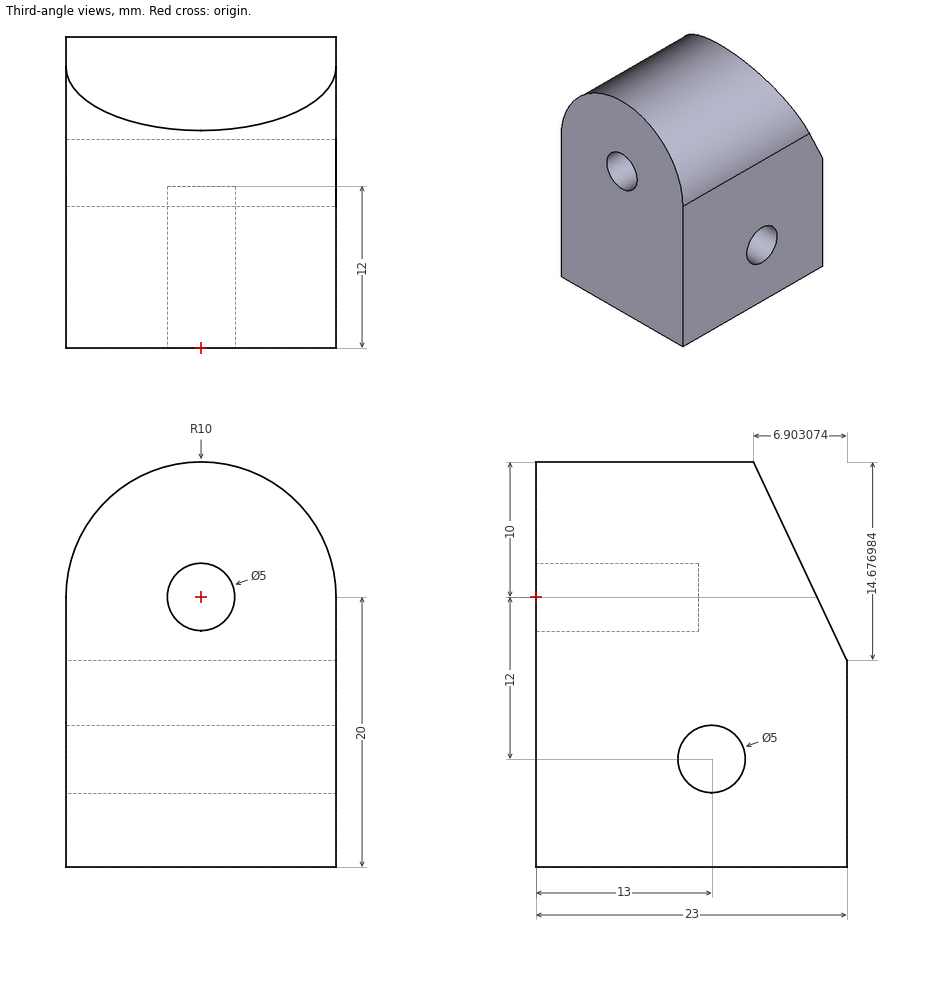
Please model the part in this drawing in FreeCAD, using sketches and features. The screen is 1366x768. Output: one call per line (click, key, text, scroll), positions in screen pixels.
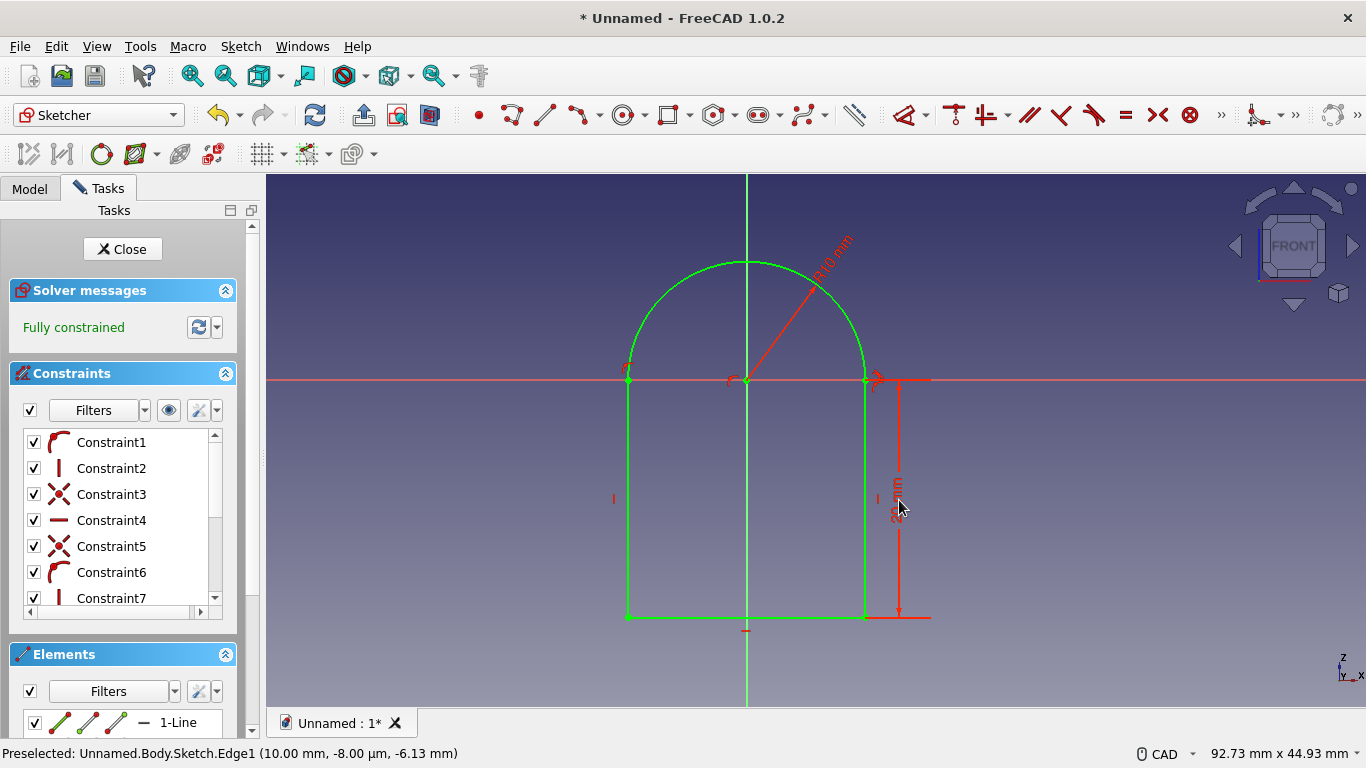
click(123, 249)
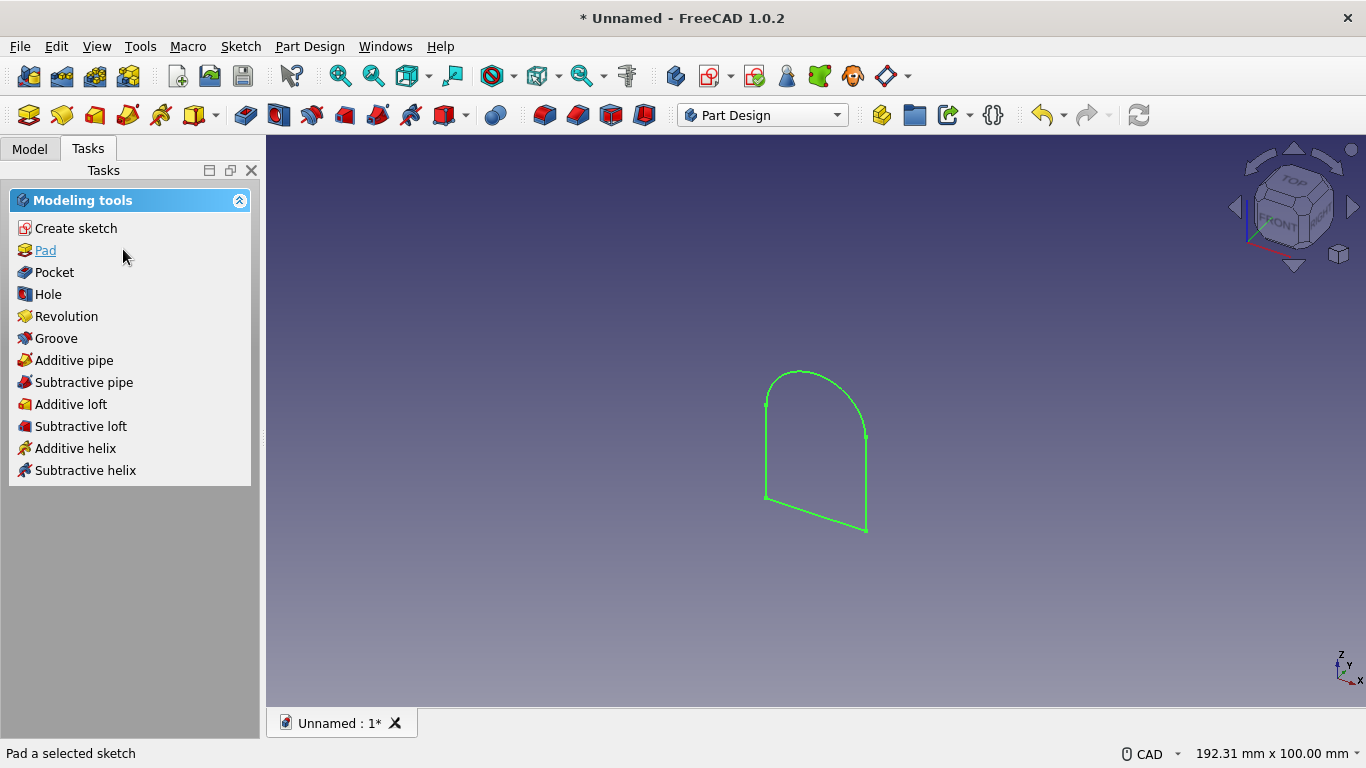
click(29, 116)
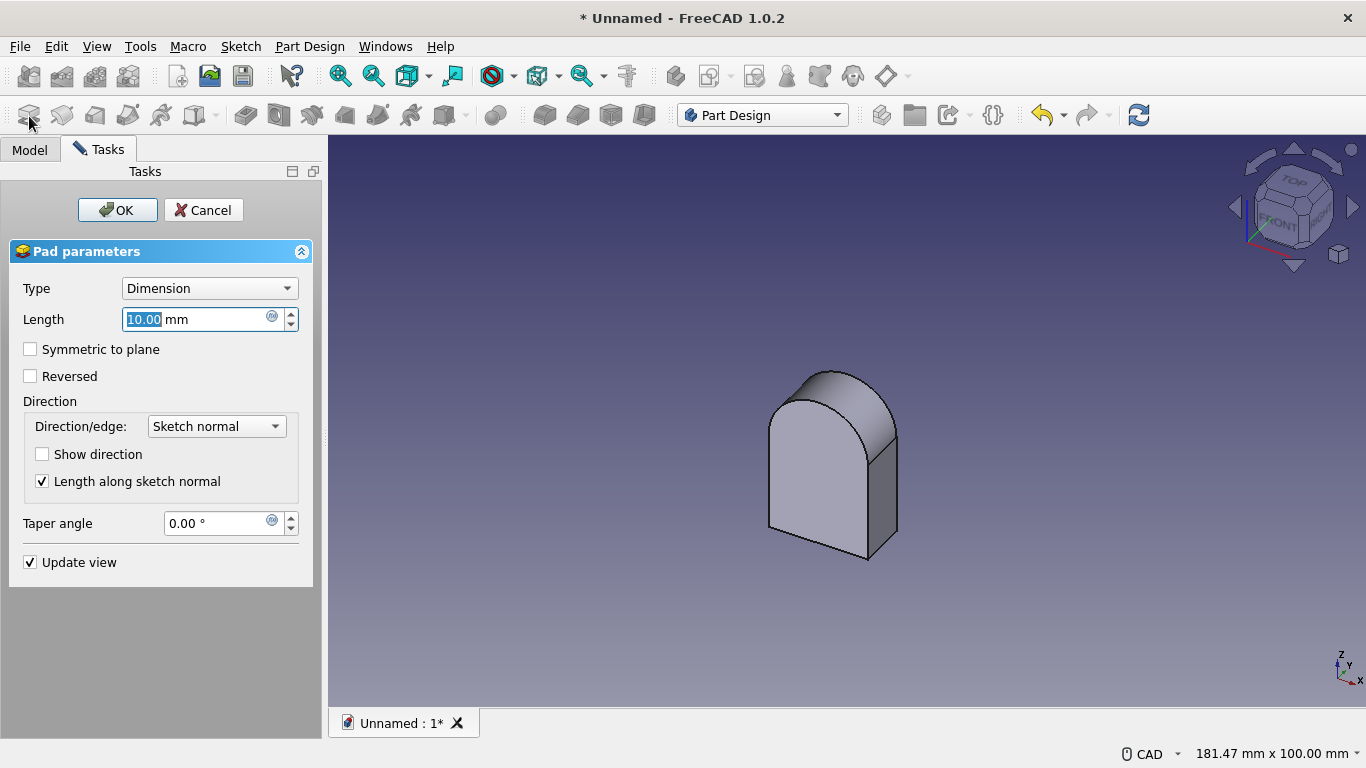
text(23)
key(Tab)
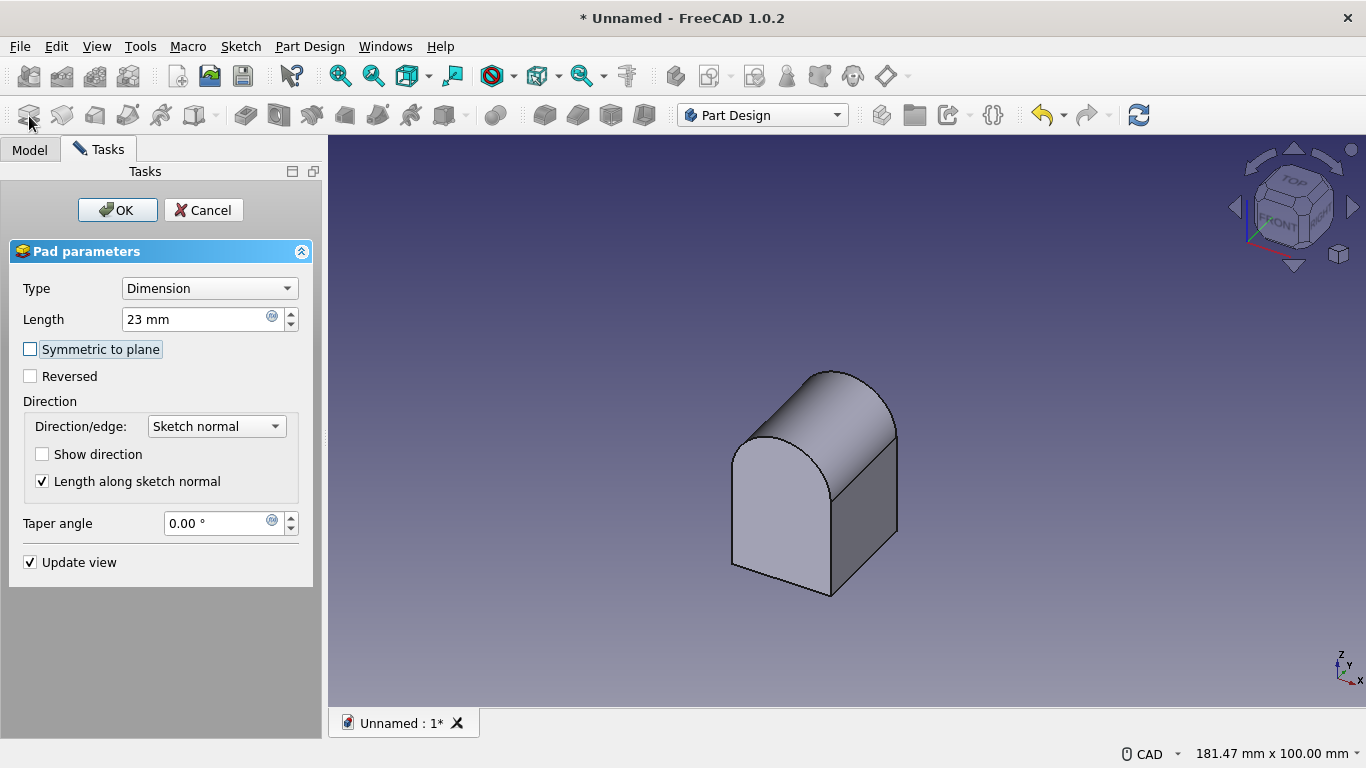
click(31, 376)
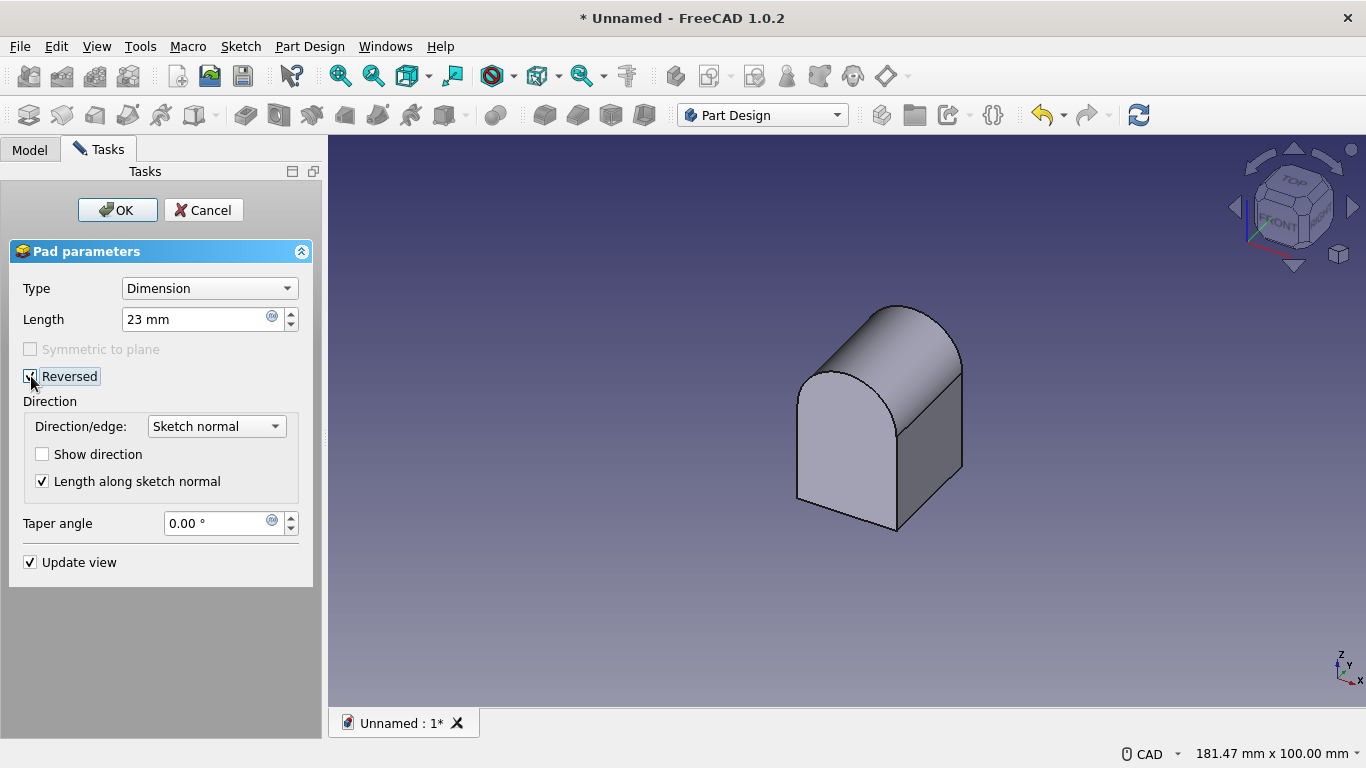
click(118, 210)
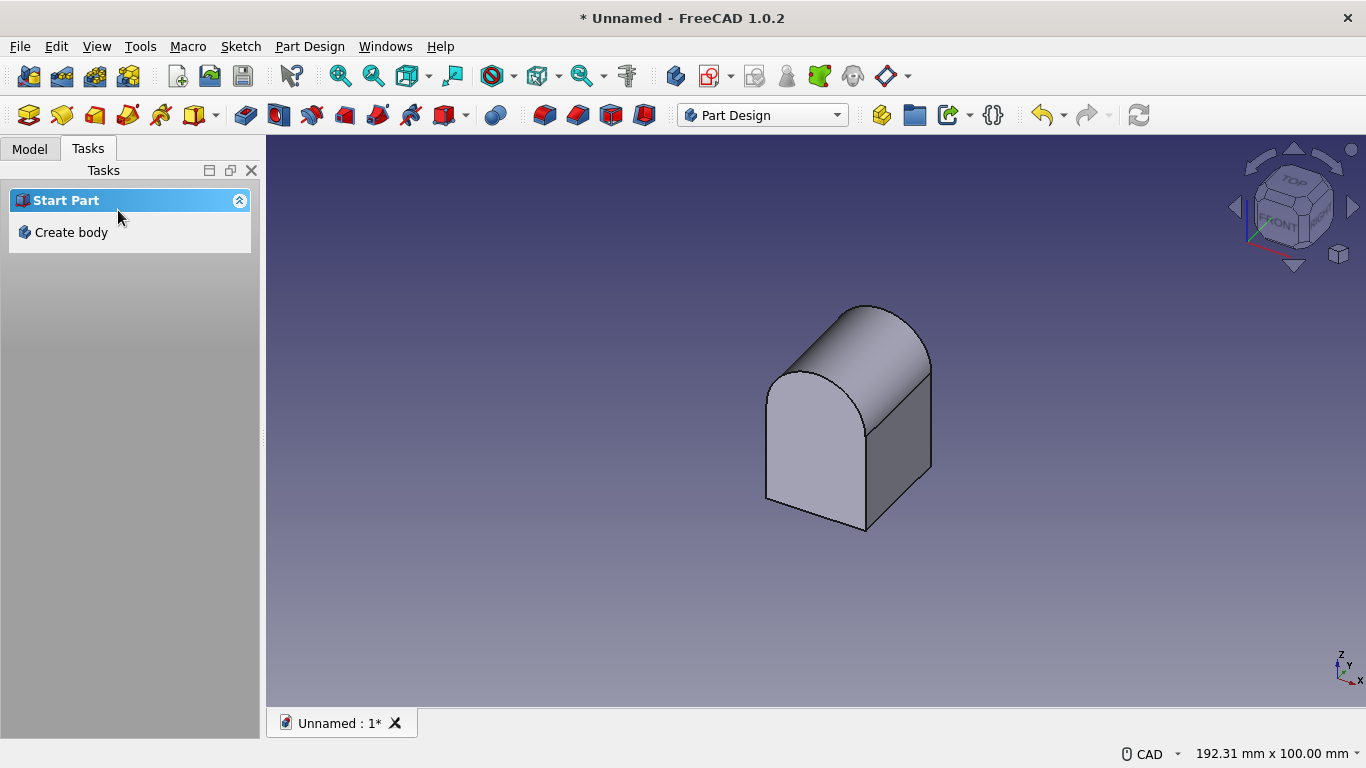
click(341, 76)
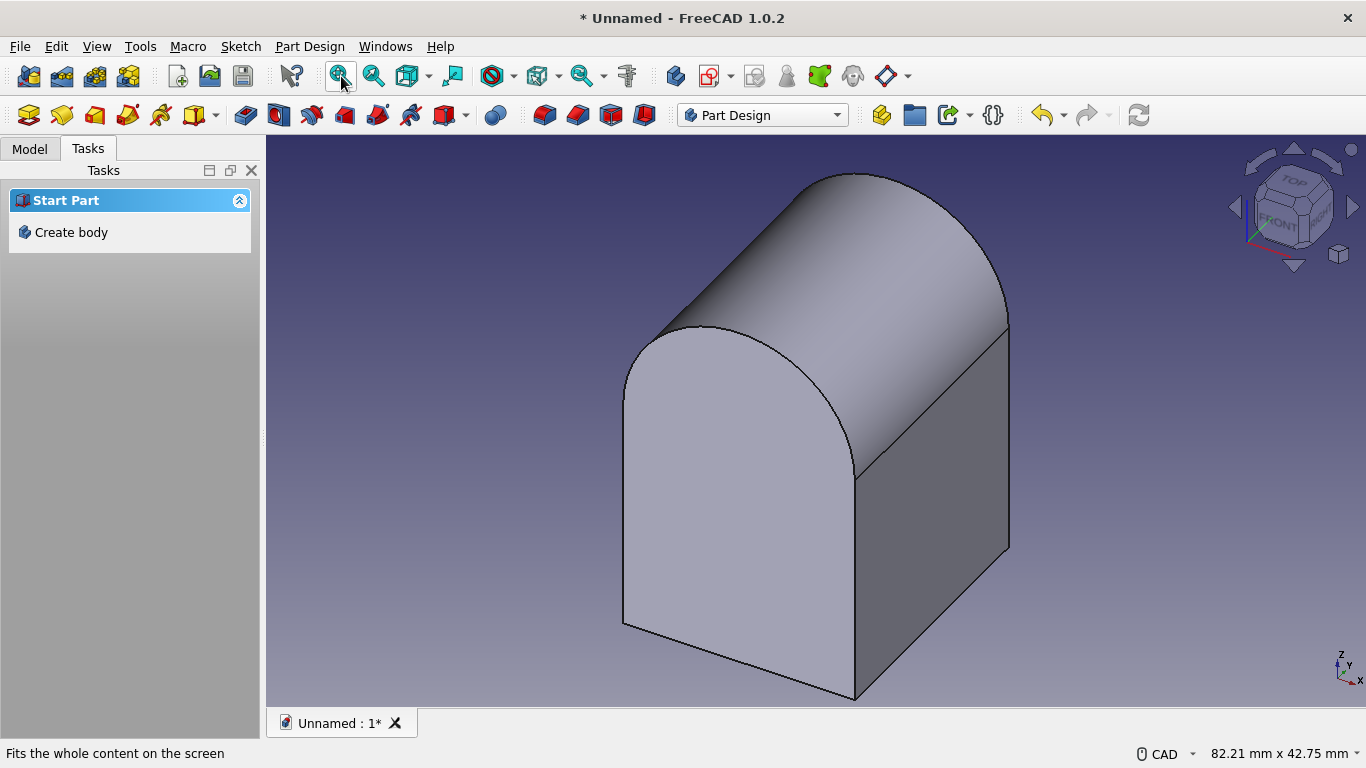
click(708, 76)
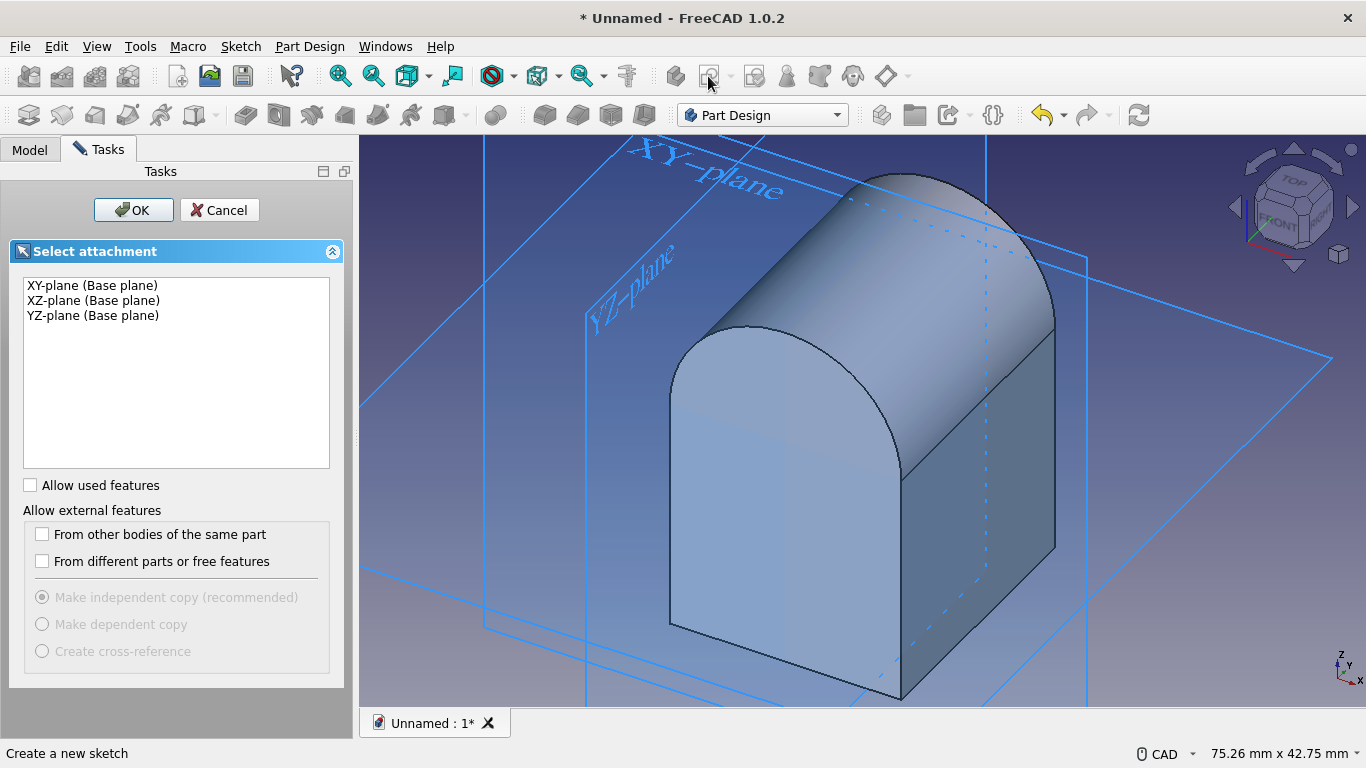
click(84, 300)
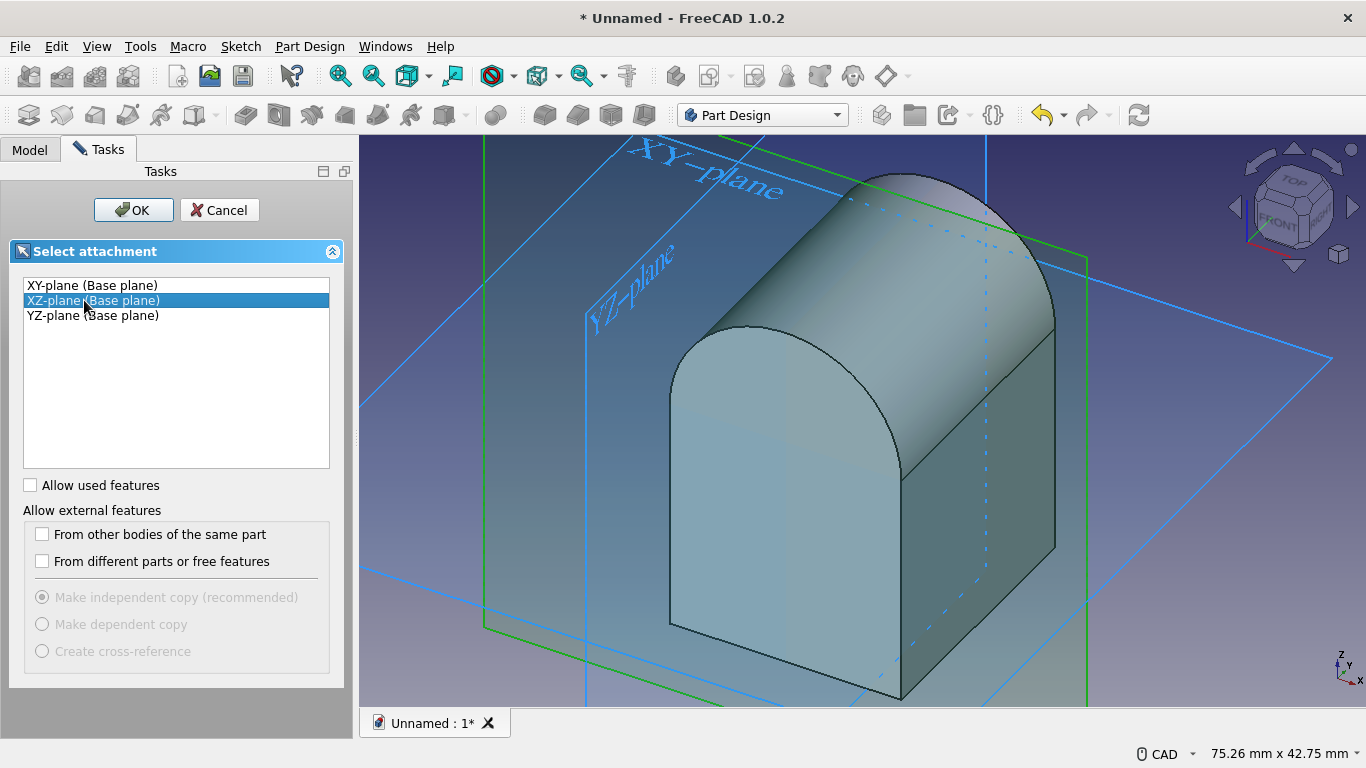
click(134, 210)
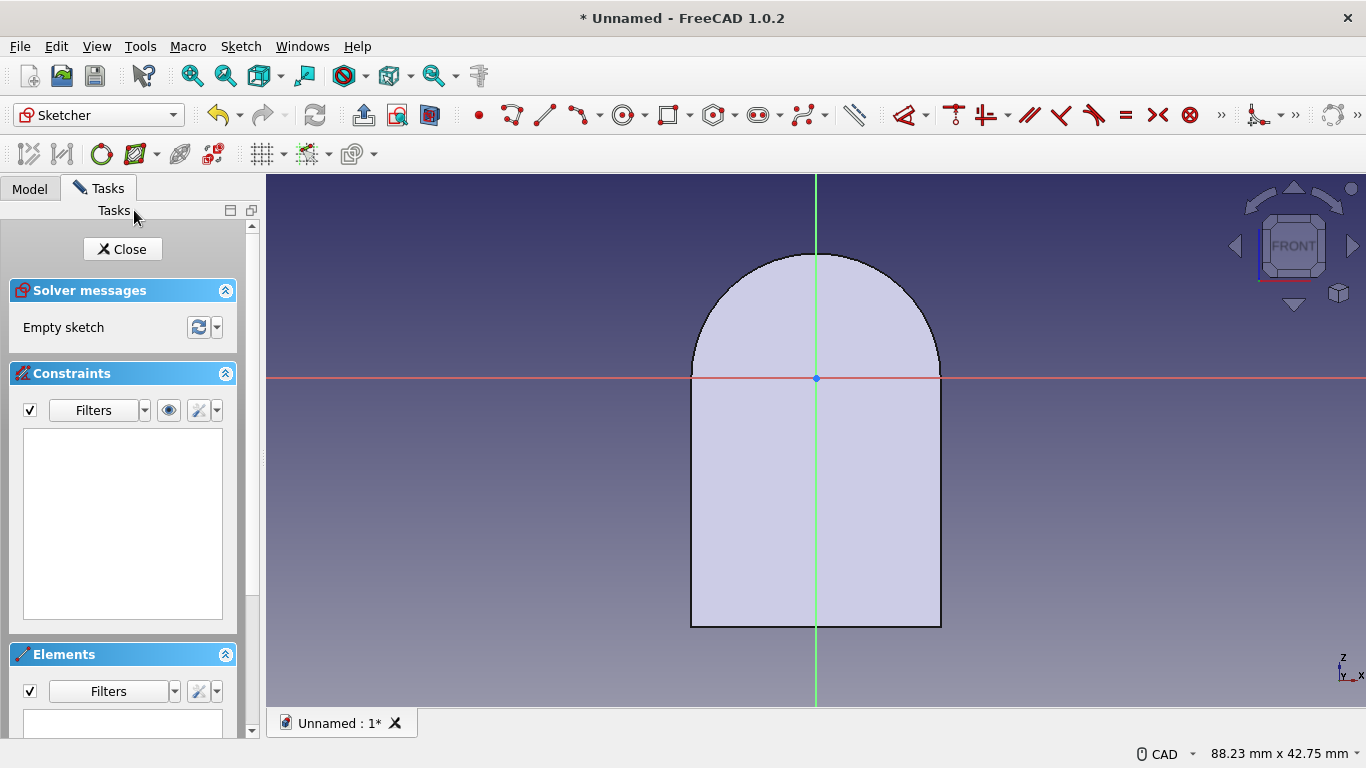
scroll(833, 362, up, 8)